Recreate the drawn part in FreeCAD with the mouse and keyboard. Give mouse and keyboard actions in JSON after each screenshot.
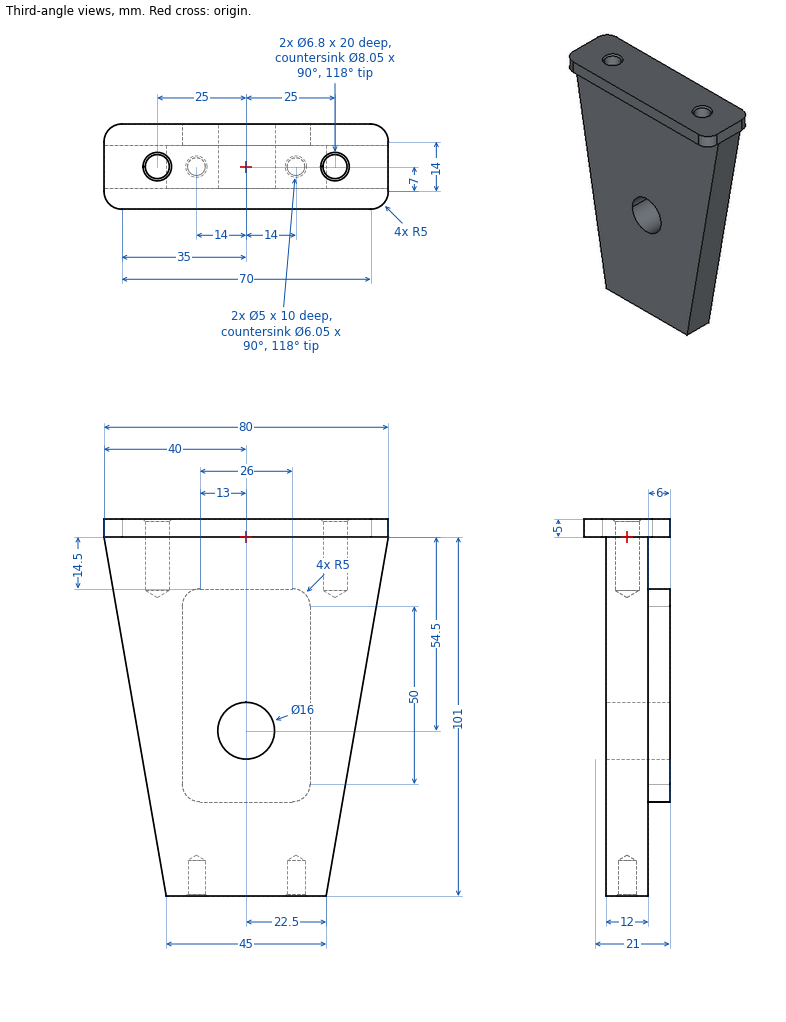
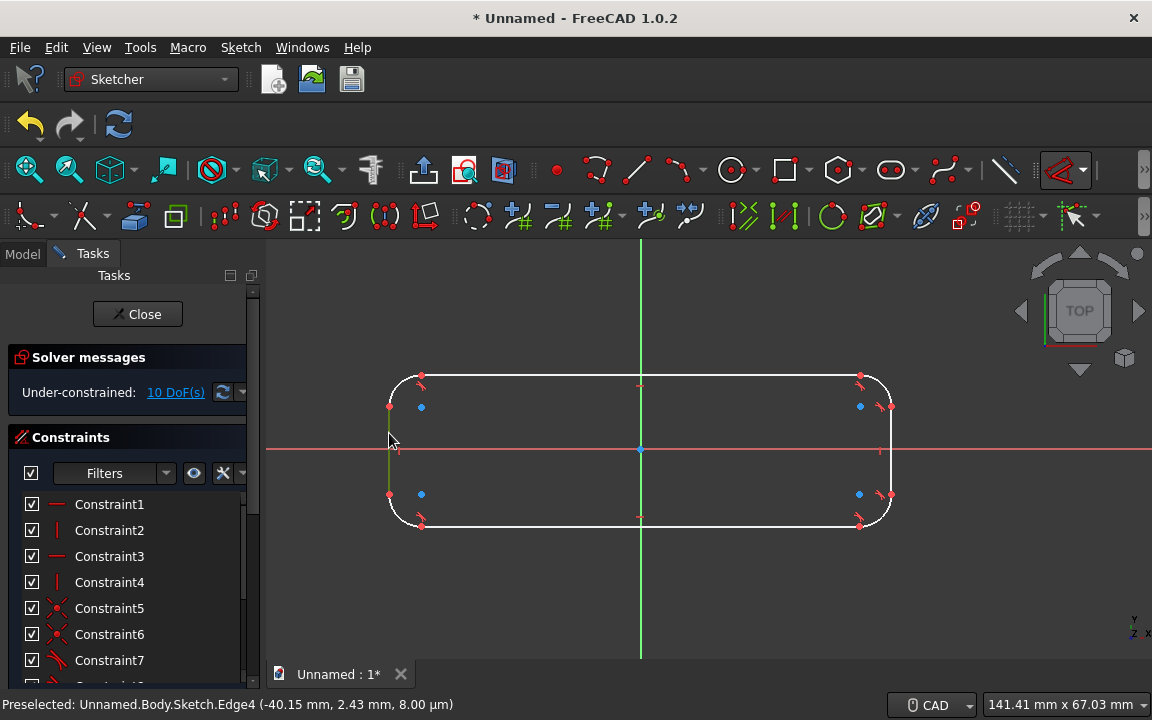
{"action": "left_click", "coordinate": [407, 379]}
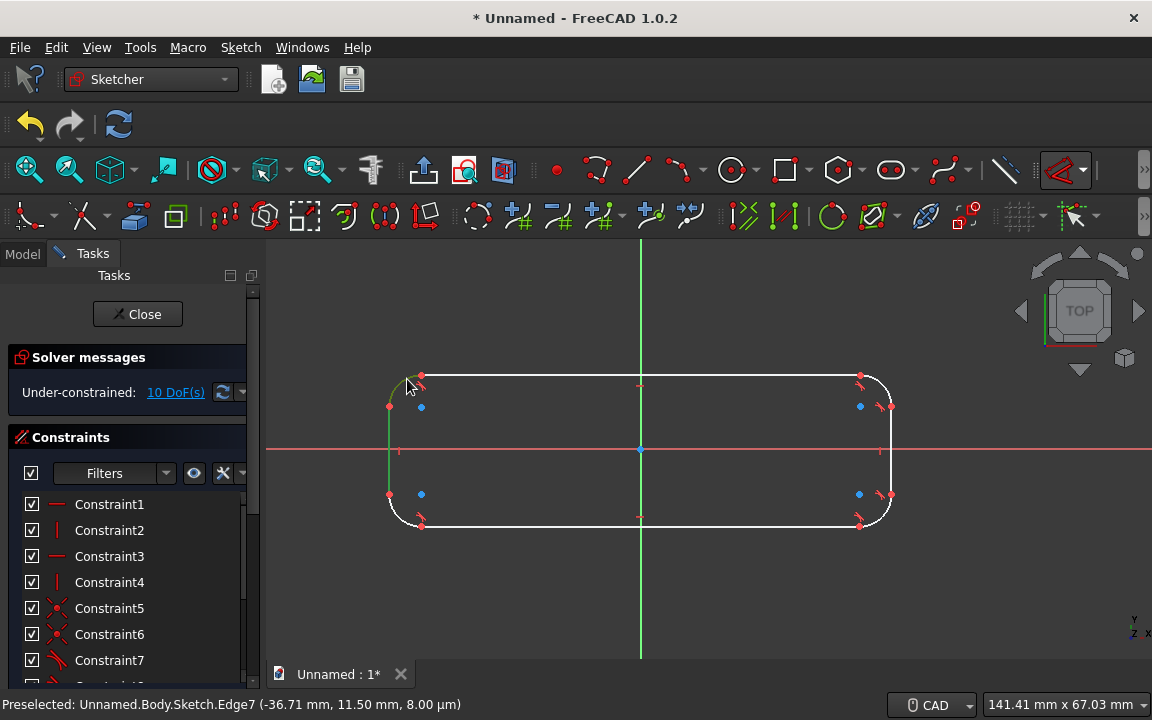
{"action": "key", "text": "t"}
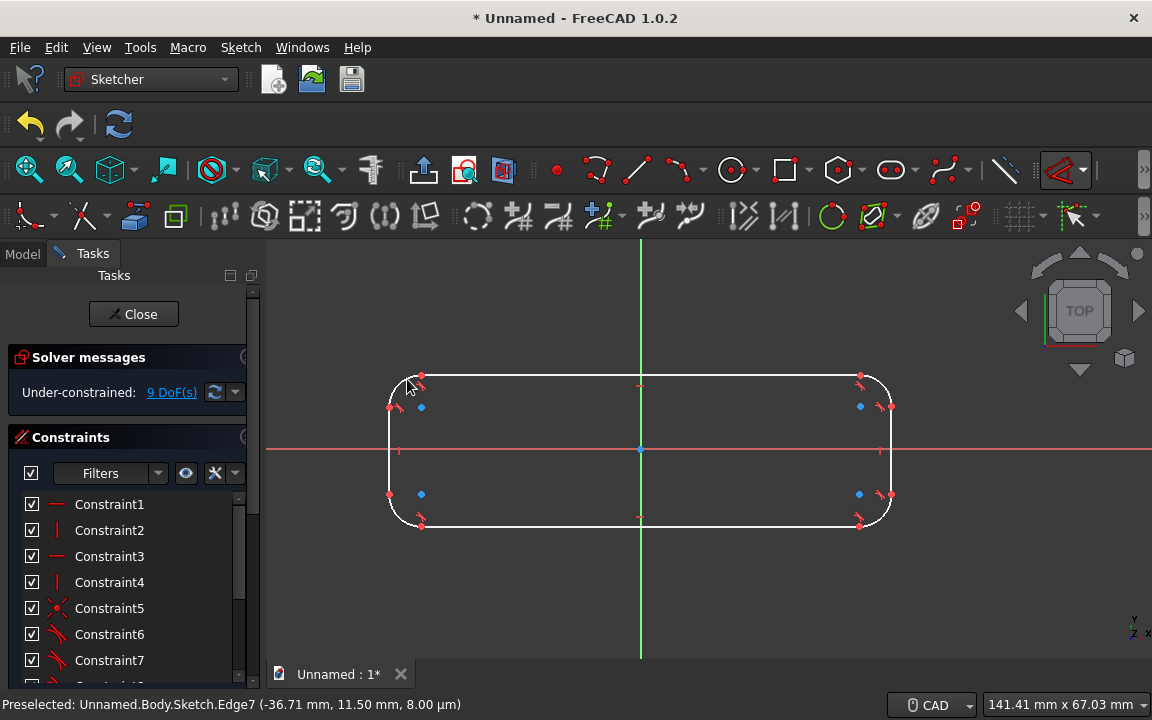
{"action": "left_click", "coordinate": [389, 434]}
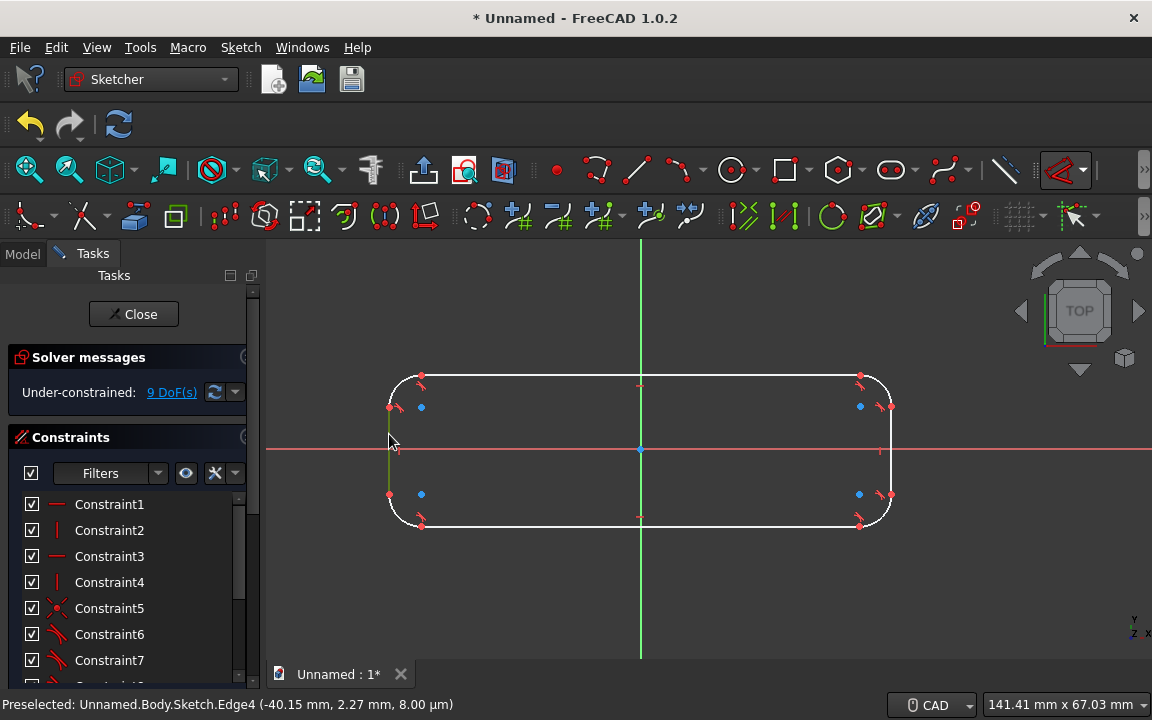
{"action": "left_click", "coordinate": [393, 509]}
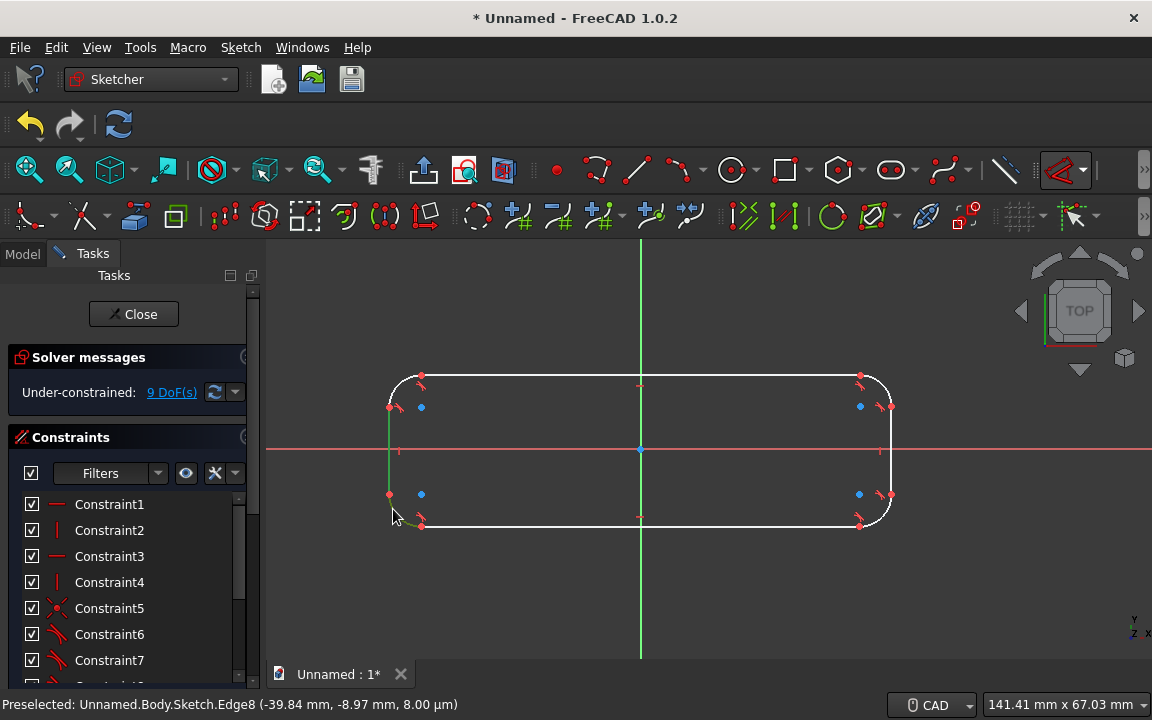
{"action": "key", "text": "t"}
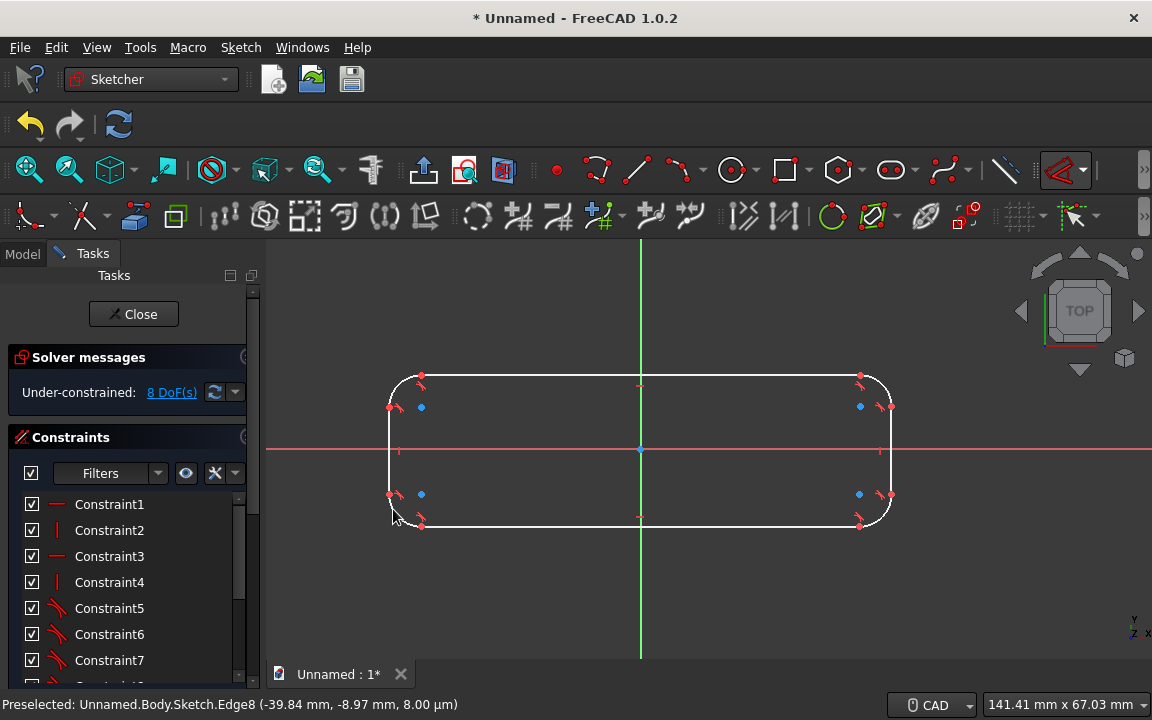
{"action": "left_click", "coordinate": [874, 523]}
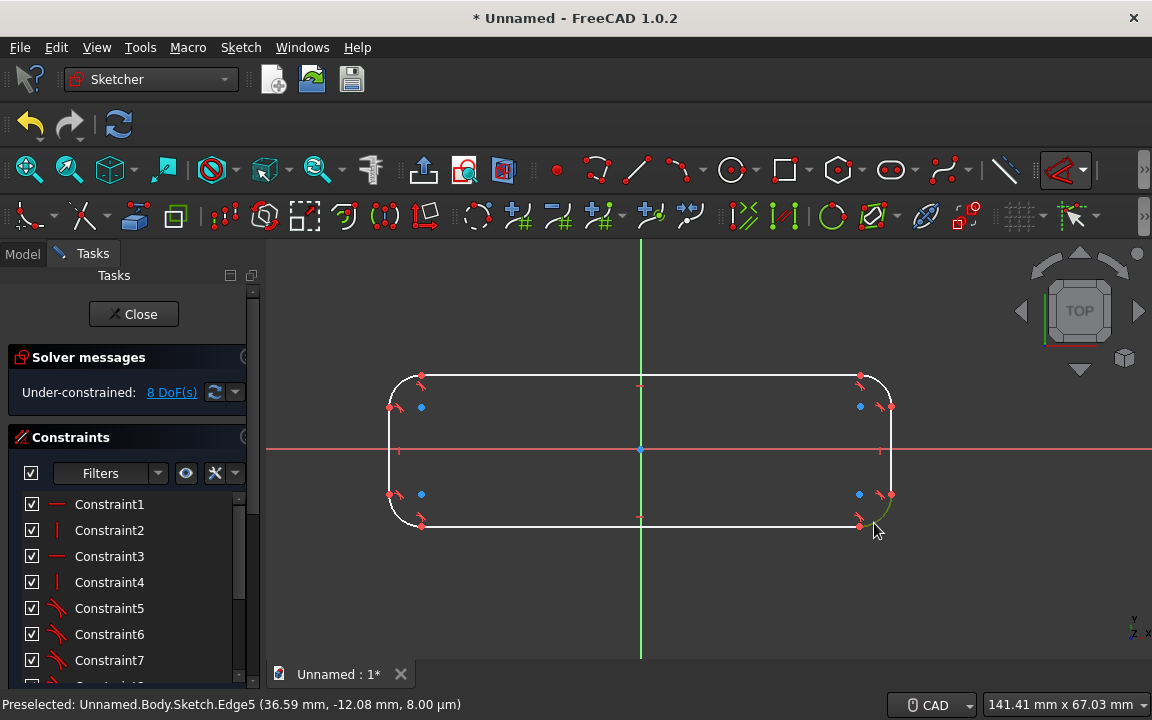
{"action": "left_click", "coordinate": [888, 392]}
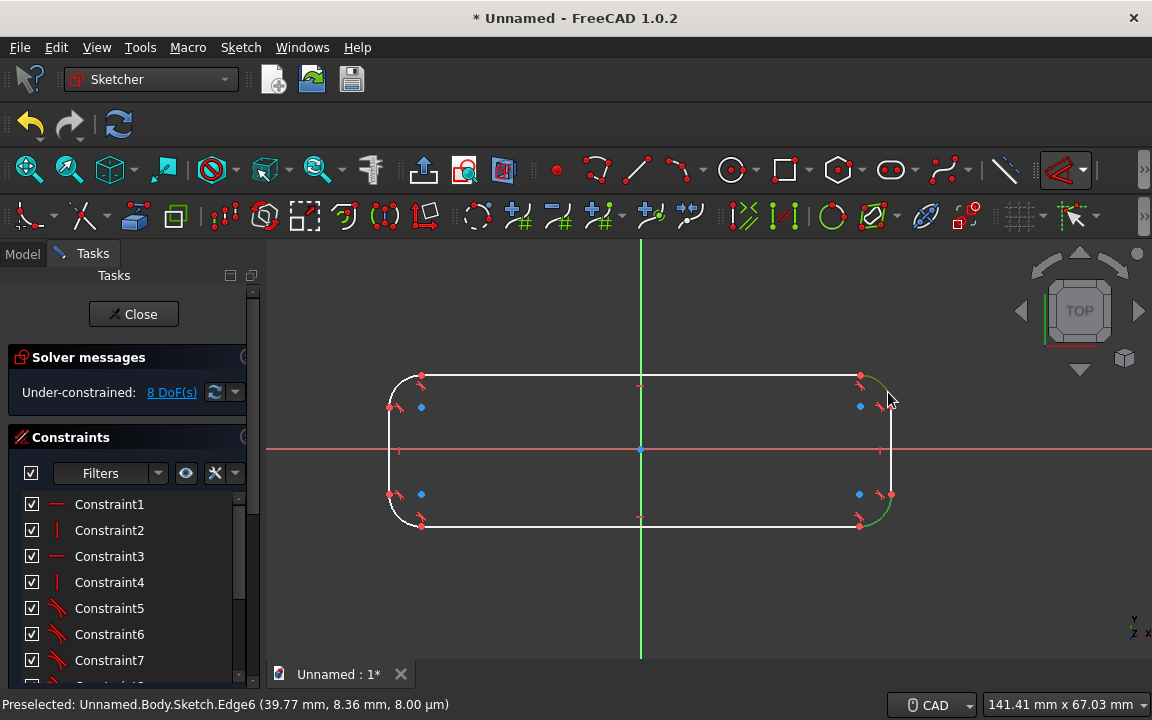
{"action": "left_click", "coordinate": [407, 379]}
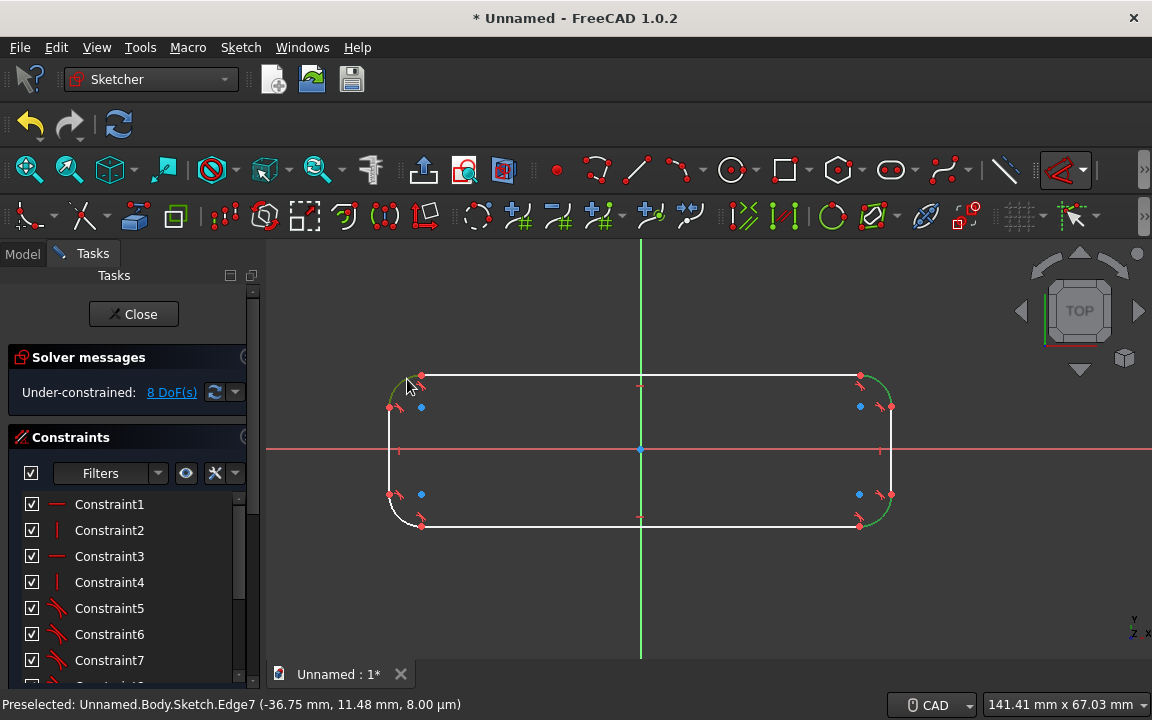
{"action": "left_click", "coordinate": [393, 509]}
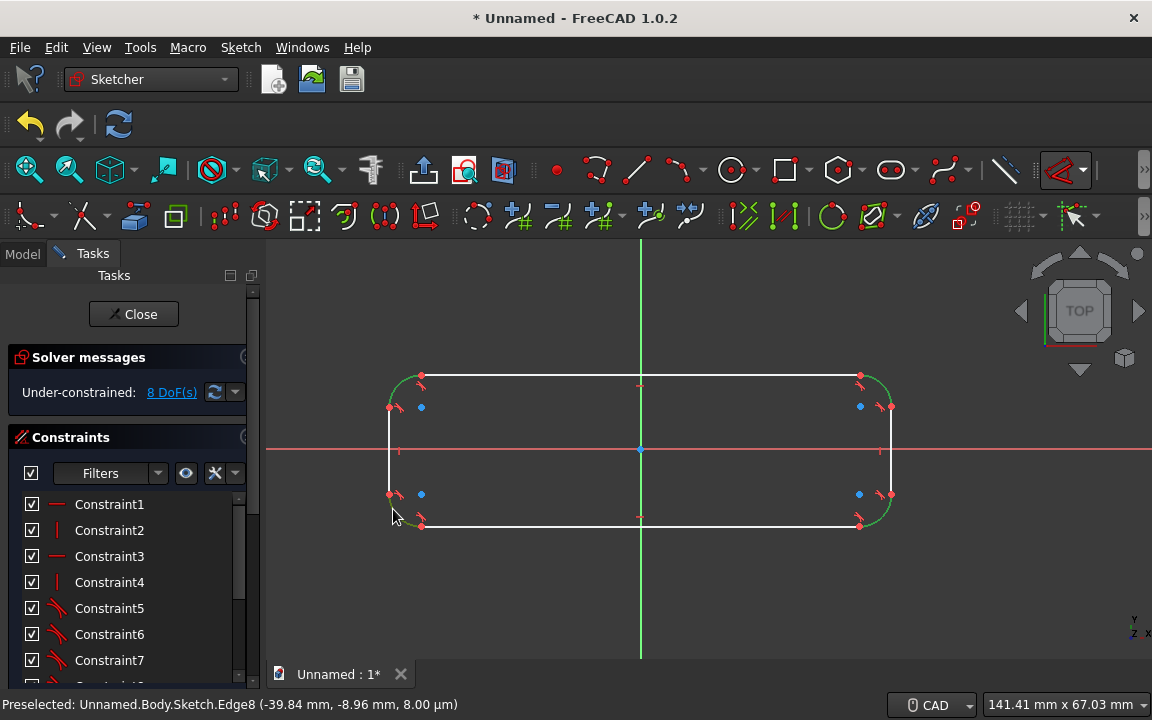
{"action": "key", "text": "e"}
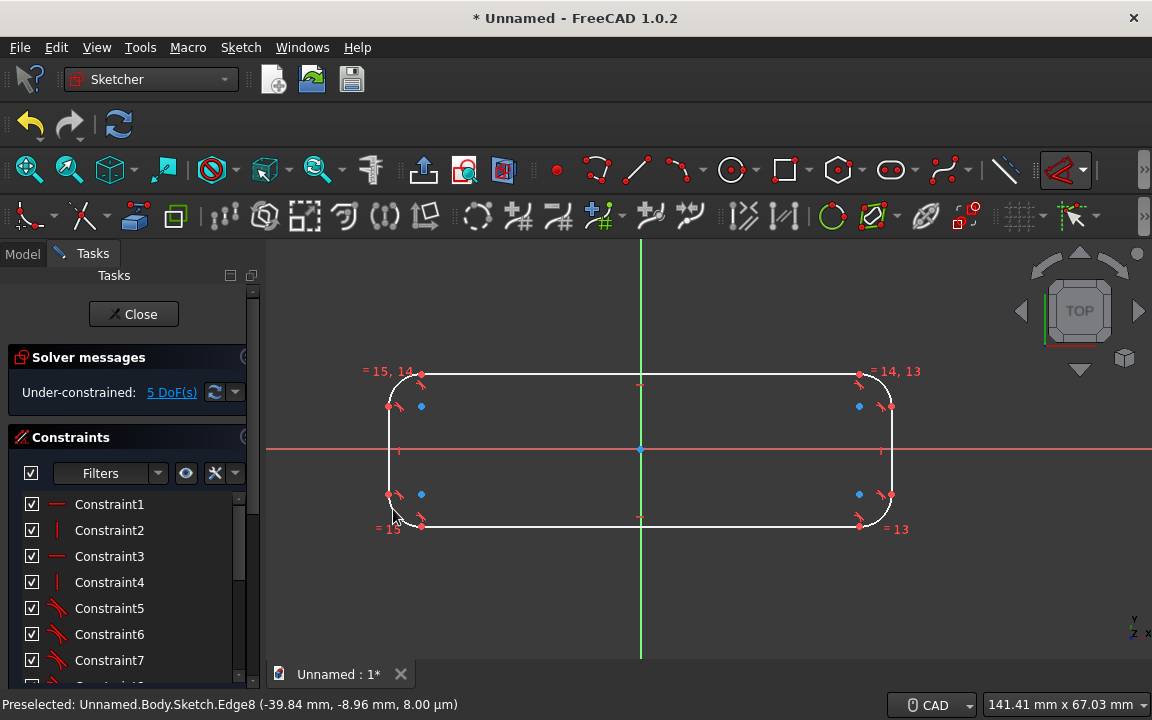
{"action": "left_click", "coordinate": [1060, 170]}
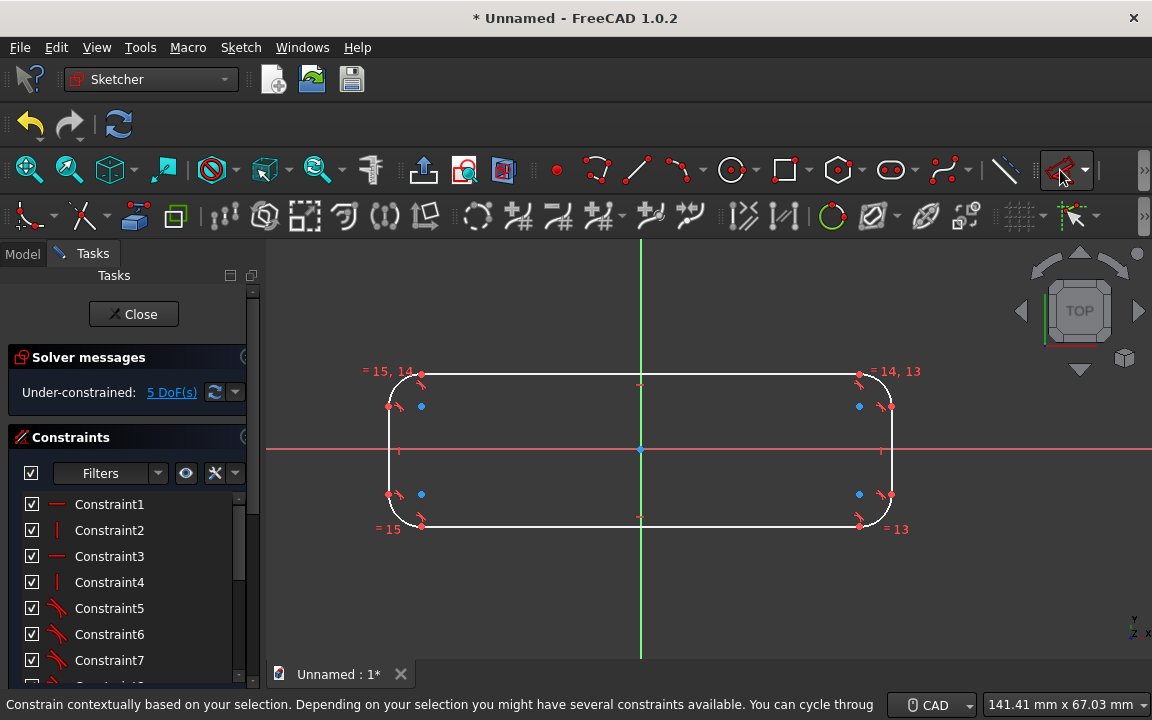
{"action": "scroll", "coordinate": [874, 523], "scroll_direction": "up", "scroll_amount": 2}